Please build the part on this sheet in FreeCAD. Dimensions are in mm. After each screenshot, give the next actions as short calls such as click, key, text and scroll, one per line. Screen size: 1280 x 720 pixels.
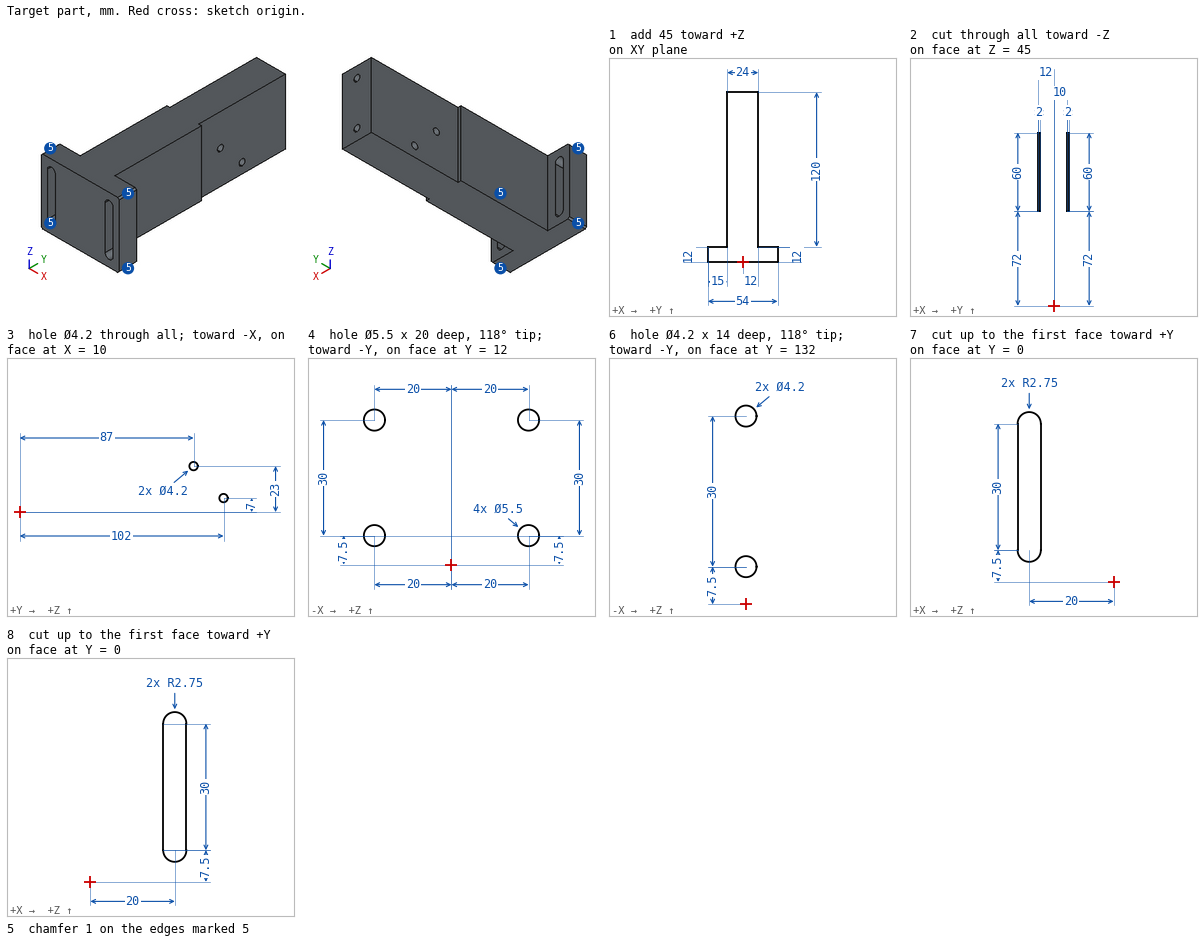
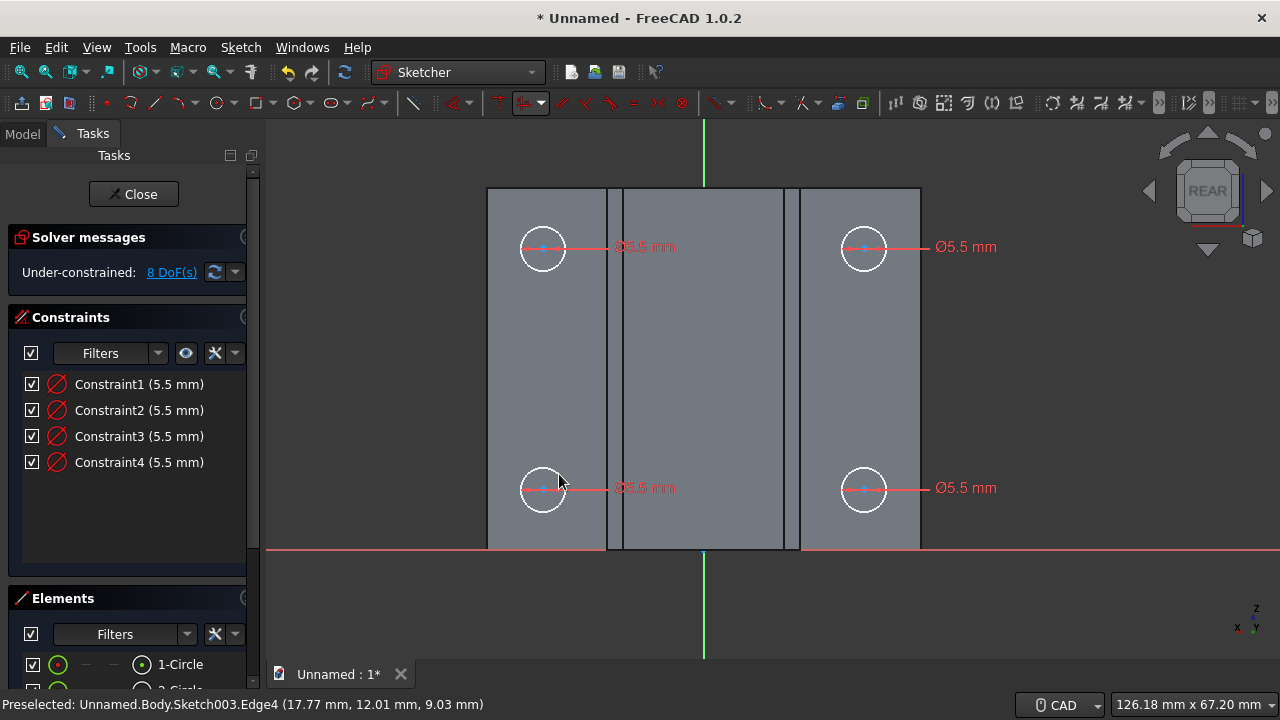
click(452, 104)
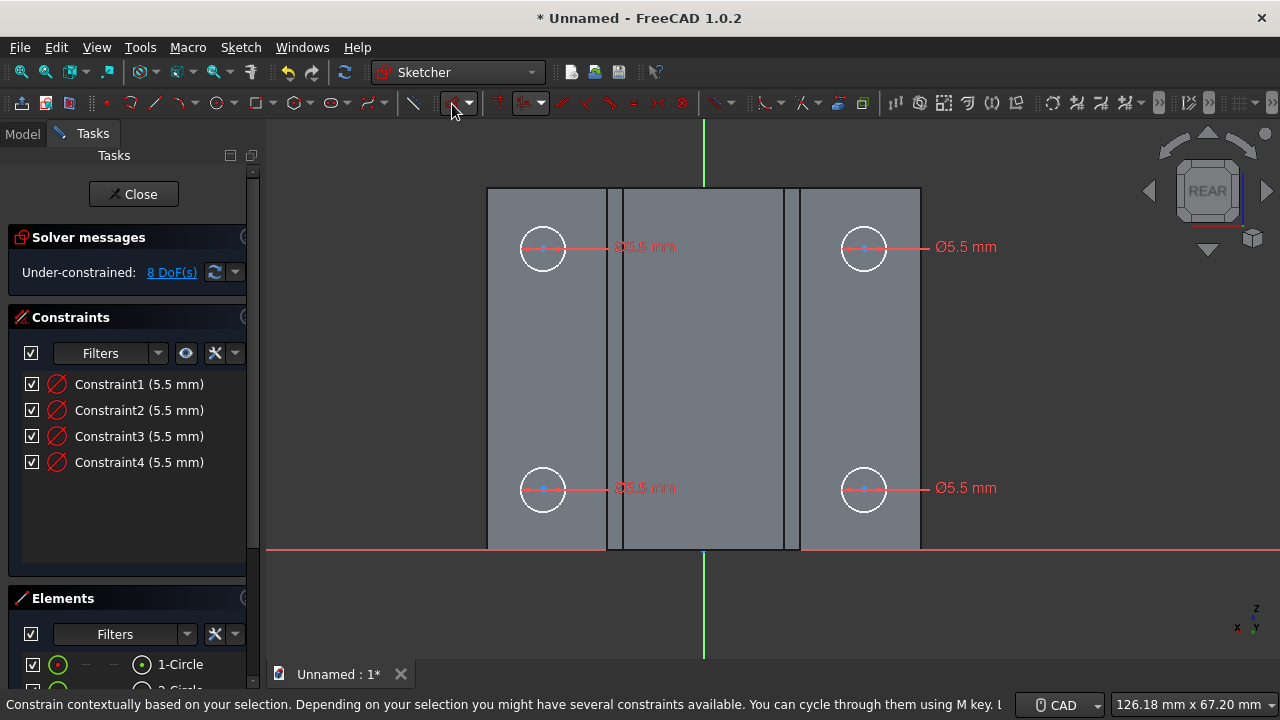
click(864, 490)
click(784, 584)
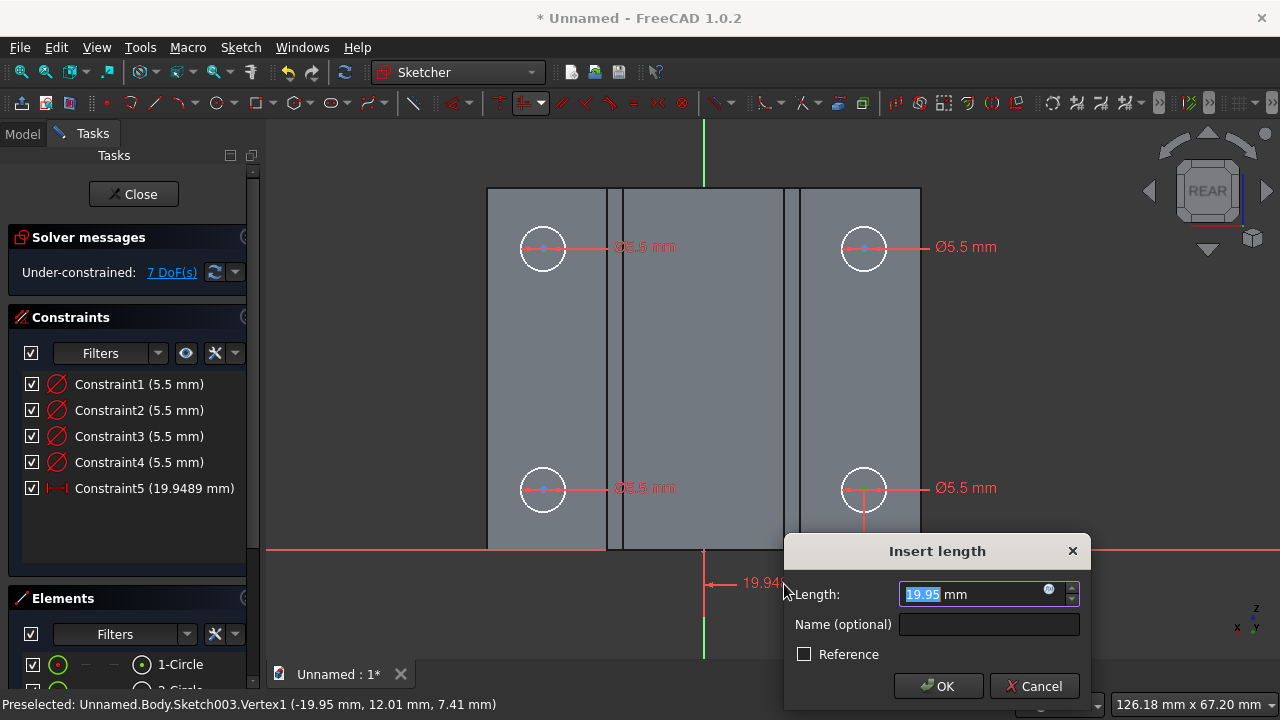
text(20)
key(Return)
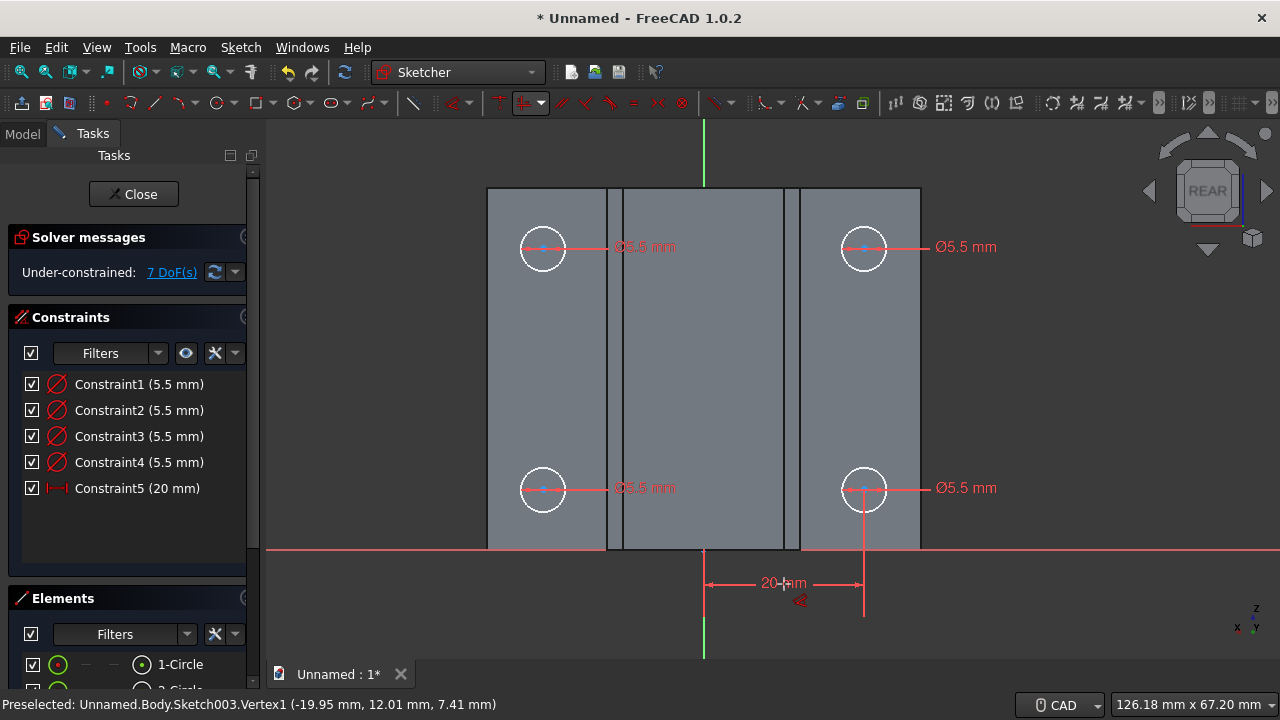
click(864, 249)
click(784, 215)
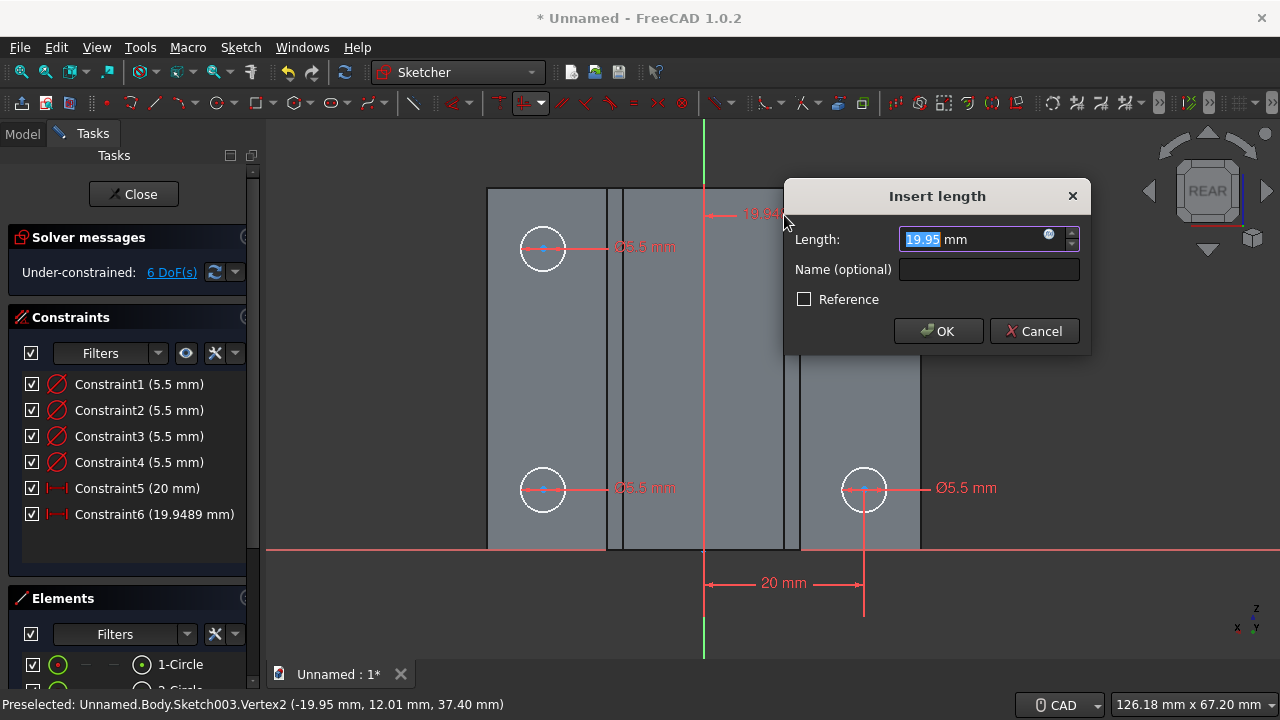
text(20)
key(Return)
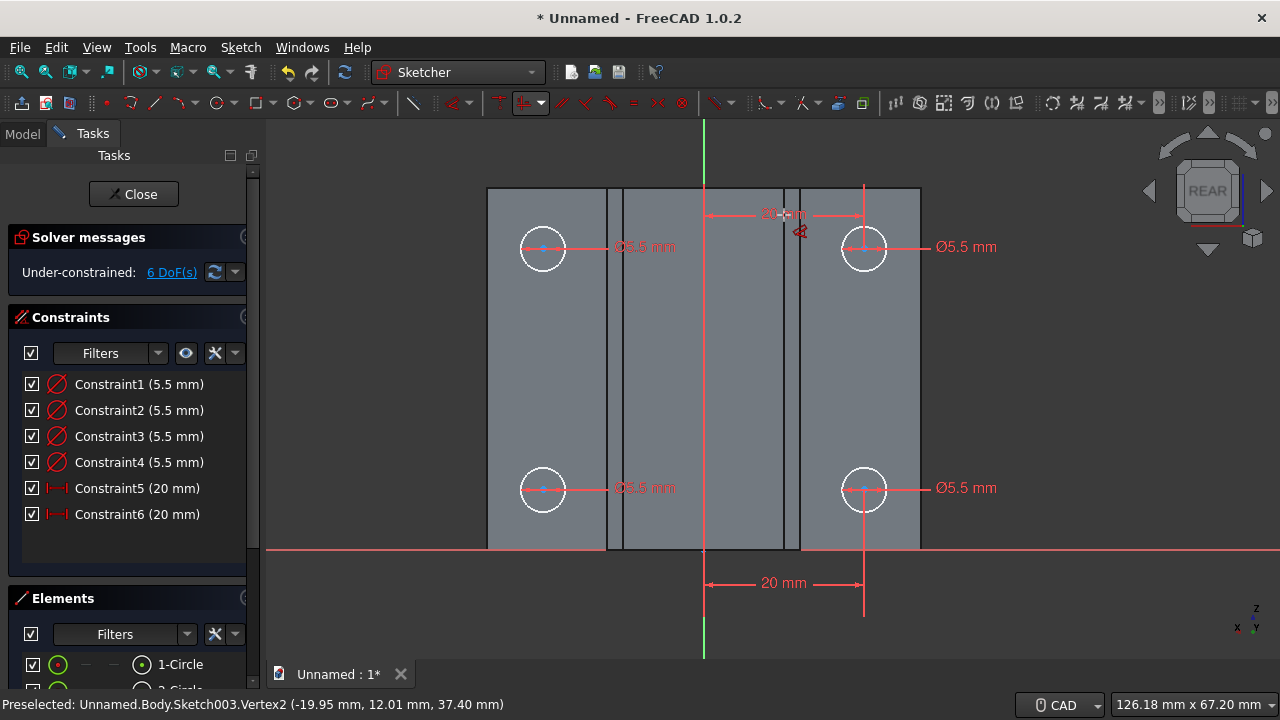
click(543, 249)
click(623, 584)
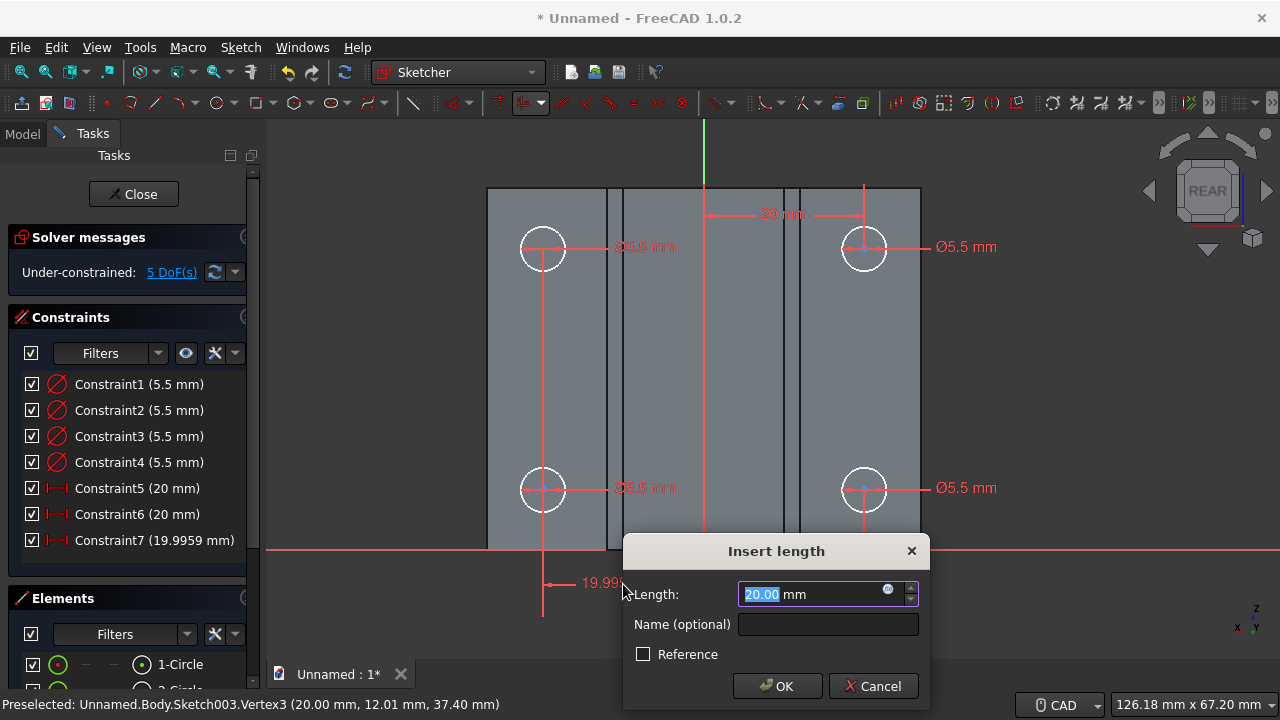
text(20)
key(Return)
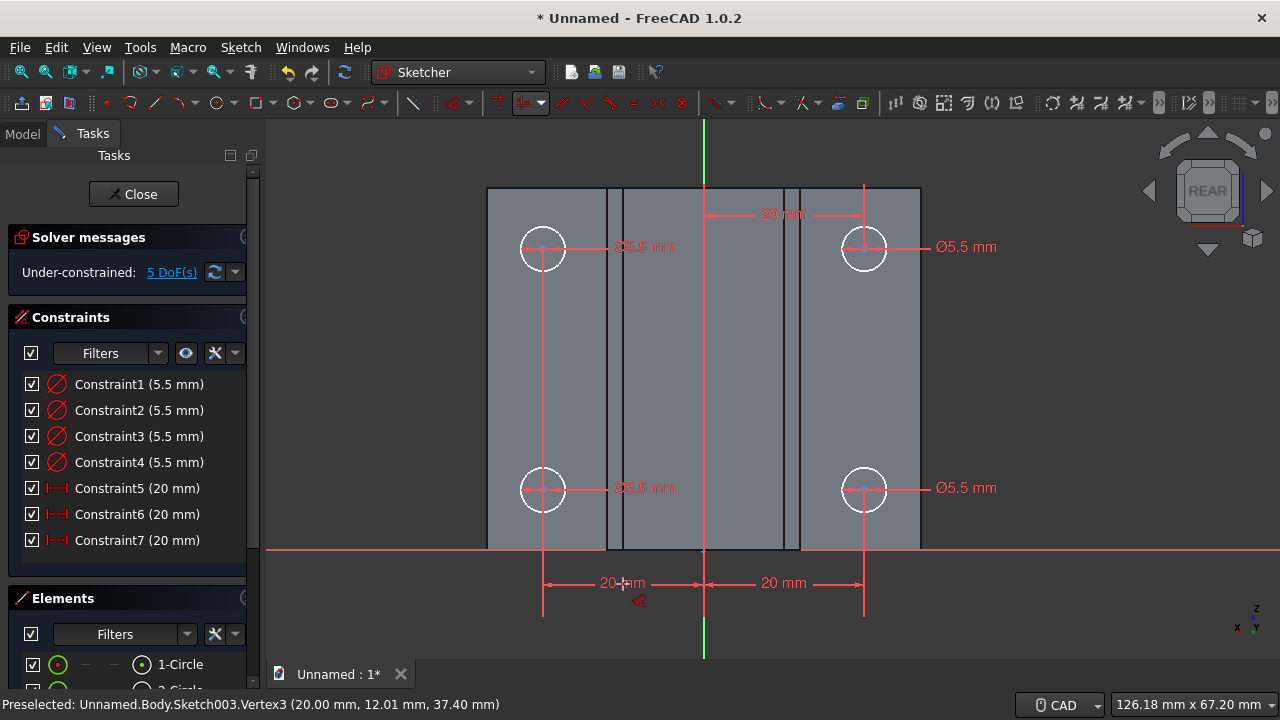
click(543, 490)
click(623, 456)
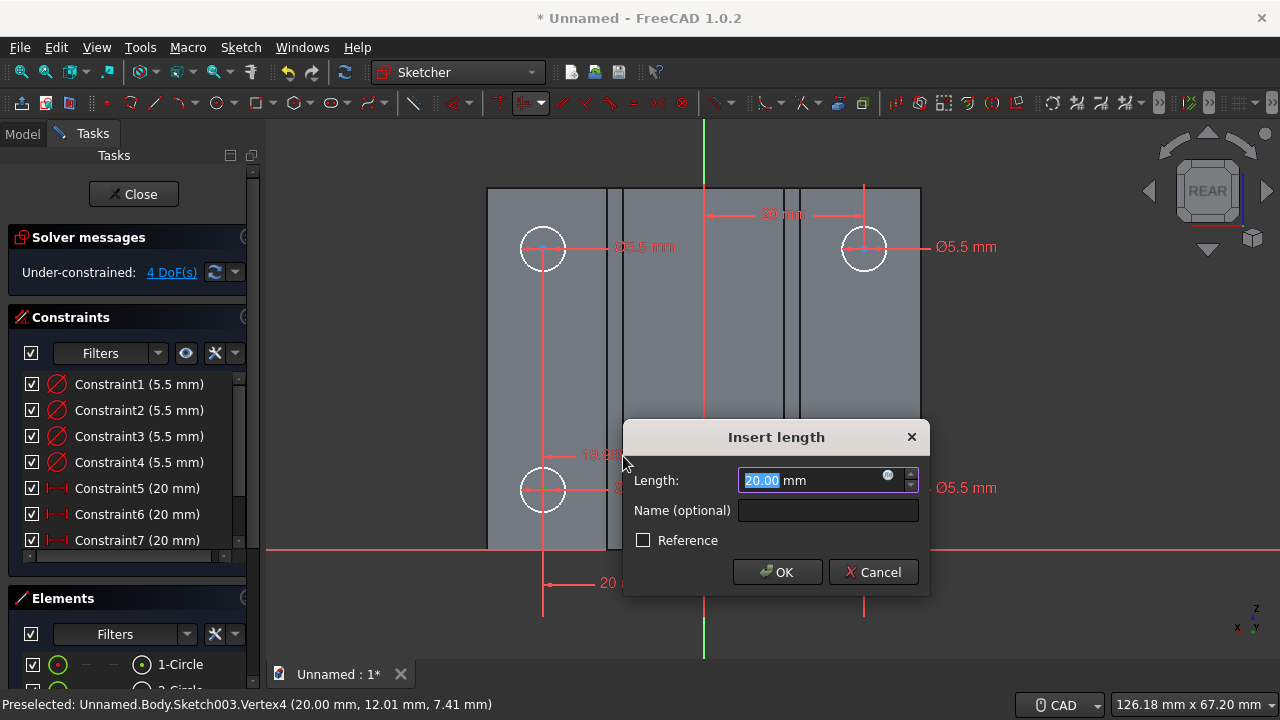
text(20)
key(Return)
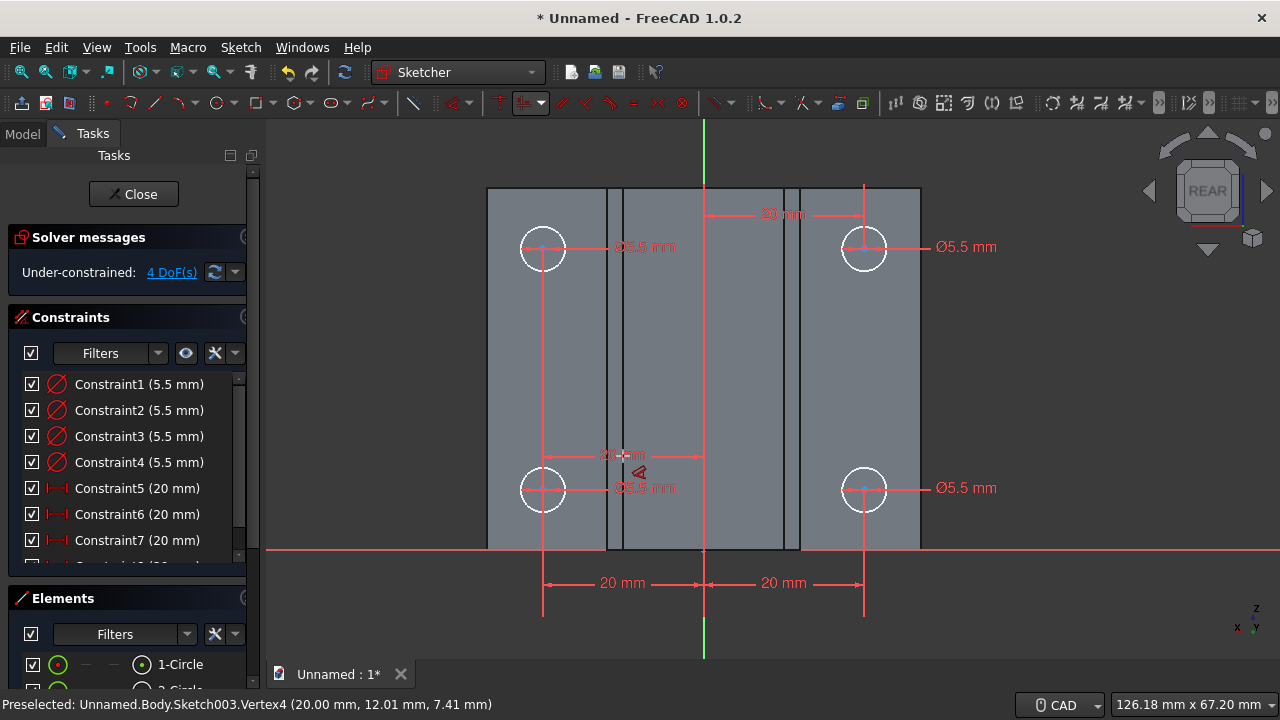
click(864, 490)
click(898, 520)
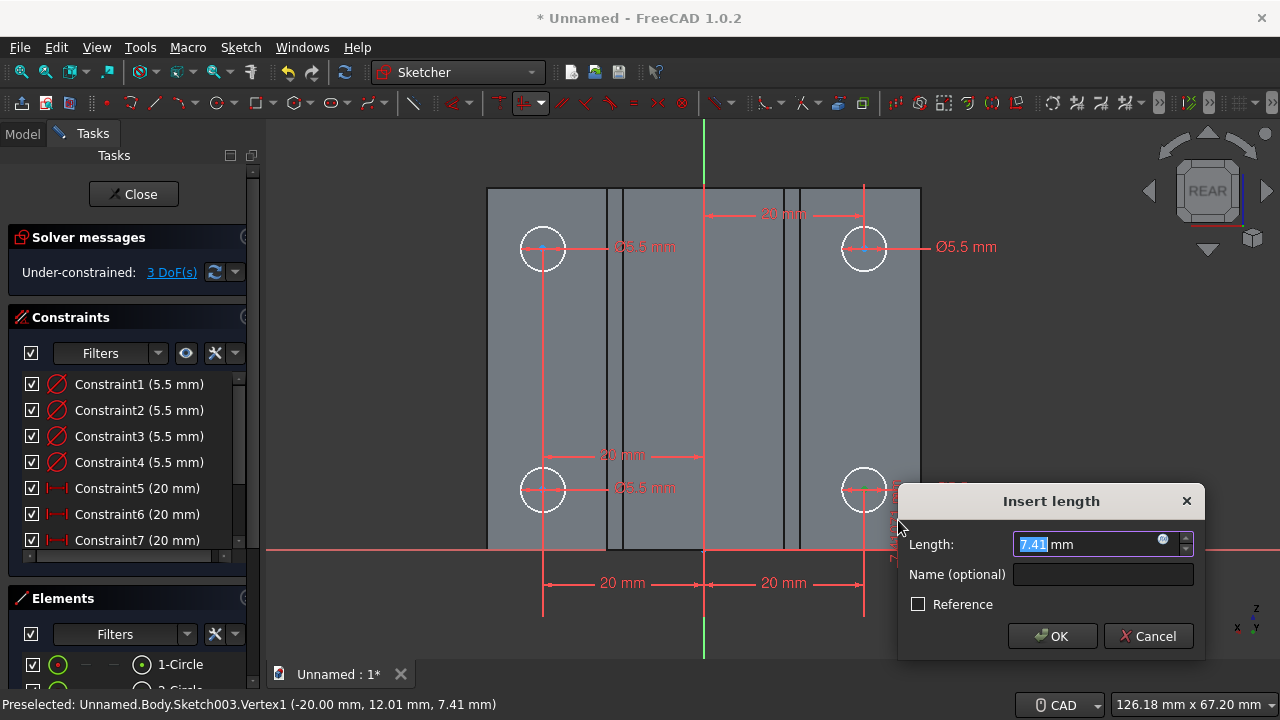
text(7.5)
key(Return)